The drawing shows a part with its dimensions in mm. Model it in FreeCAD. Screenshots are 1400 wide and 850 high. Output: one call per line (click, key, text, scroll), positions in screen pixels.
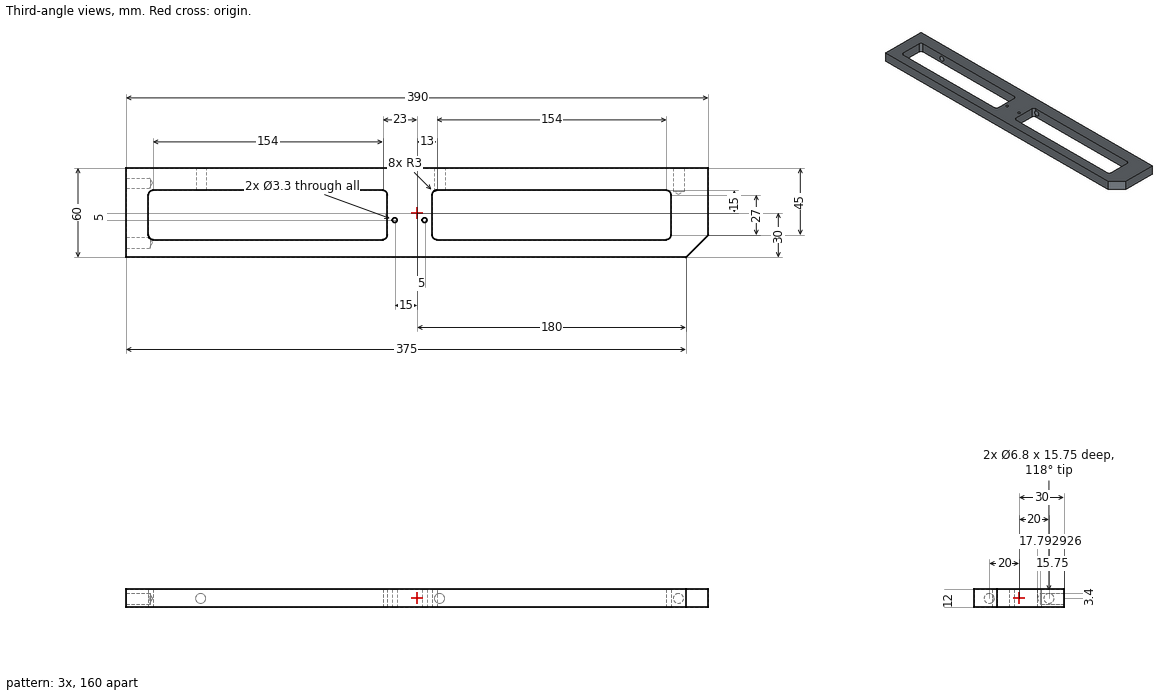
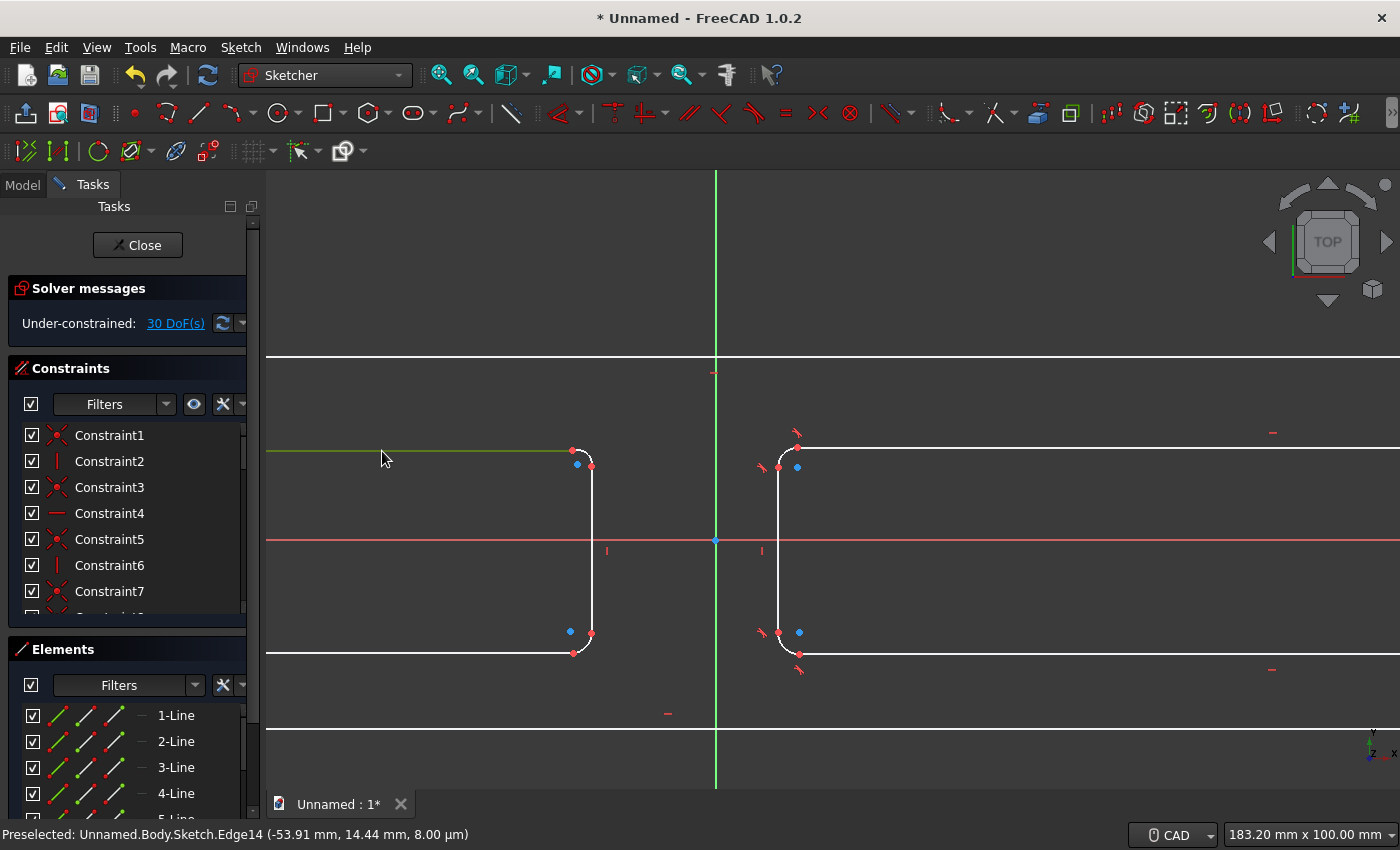
click(587, 453)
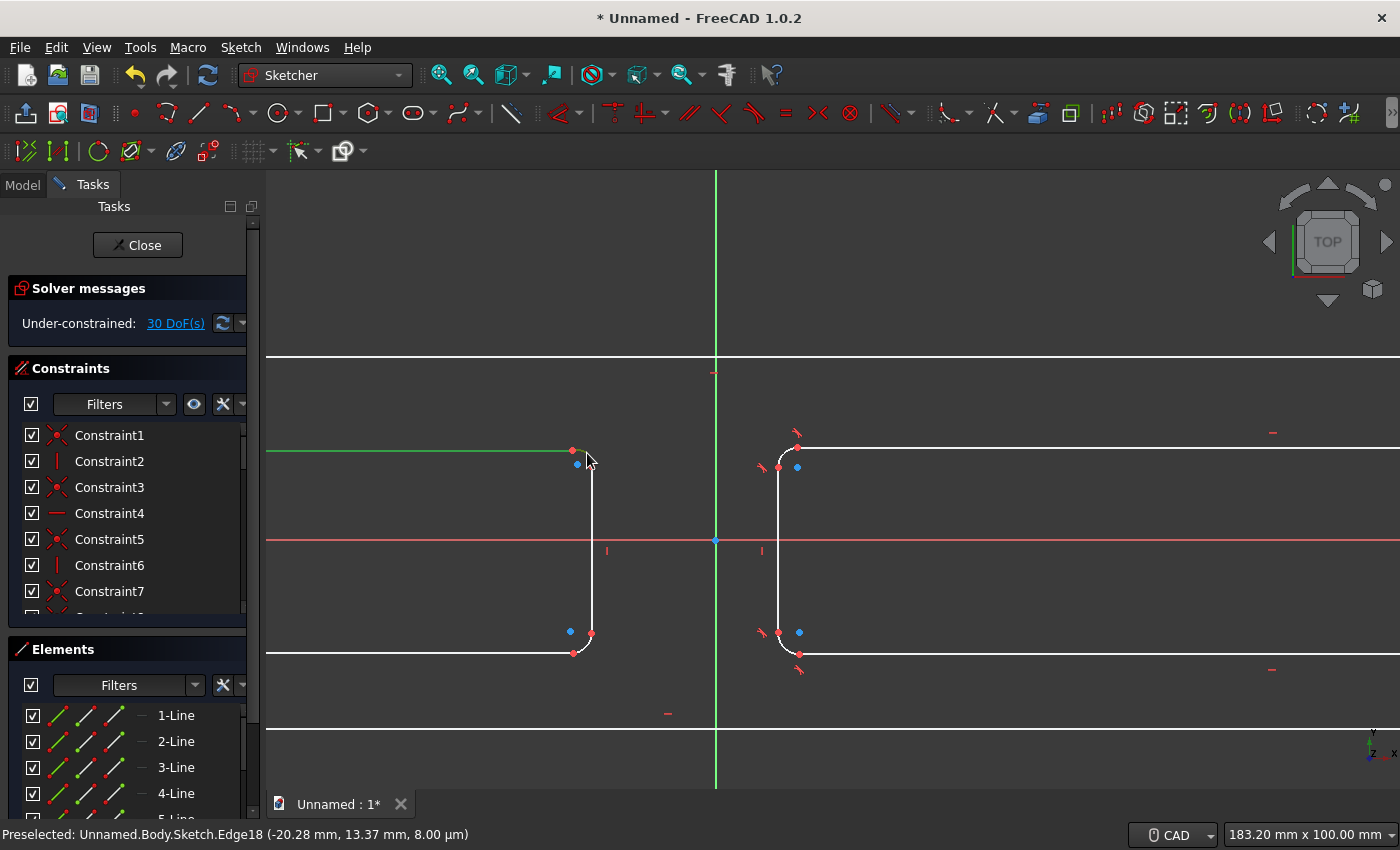
click(754, 114)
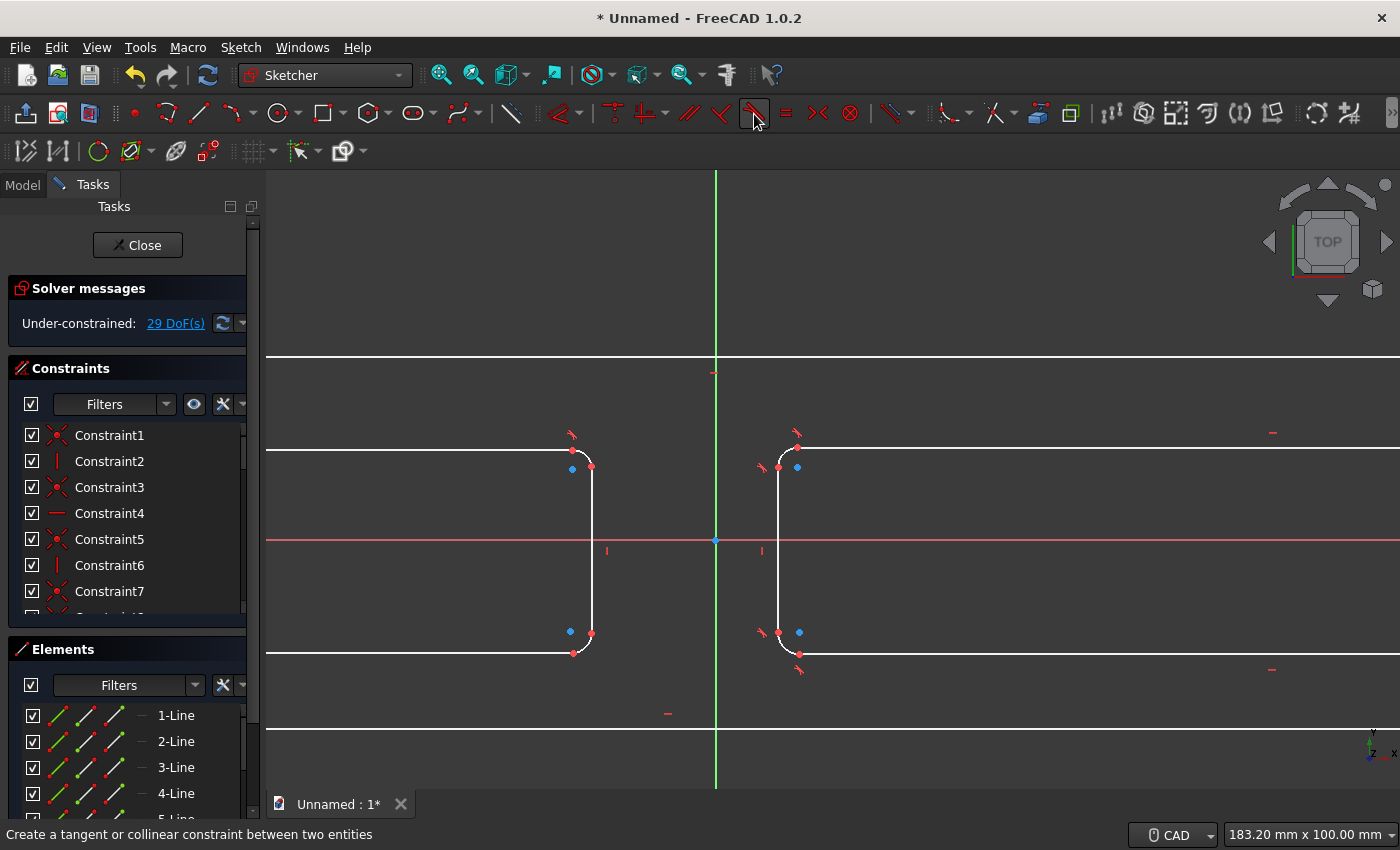
click(382, 450)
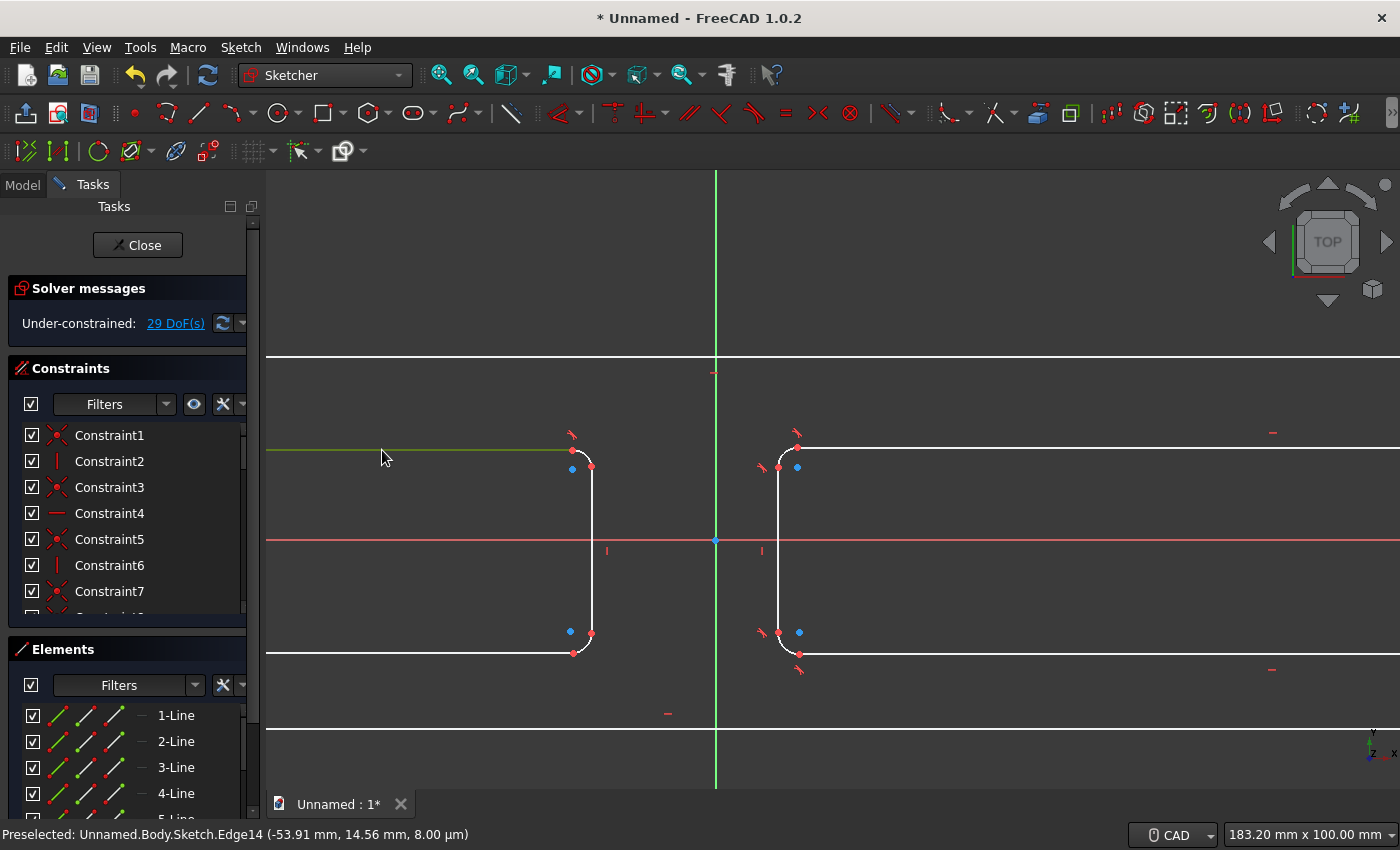
scroll(786, 453, down, 6)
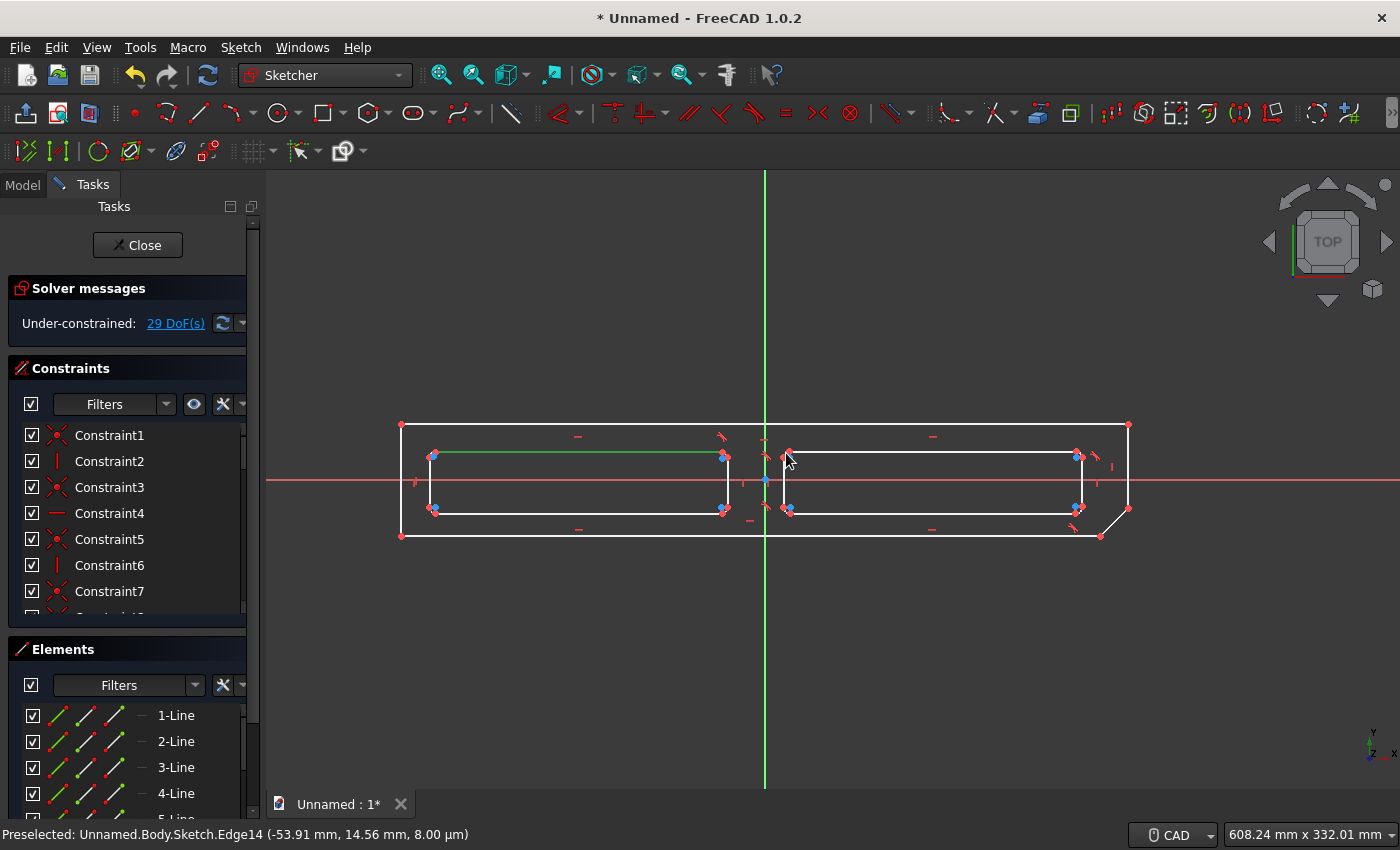
scroll(431, 454, up, 6)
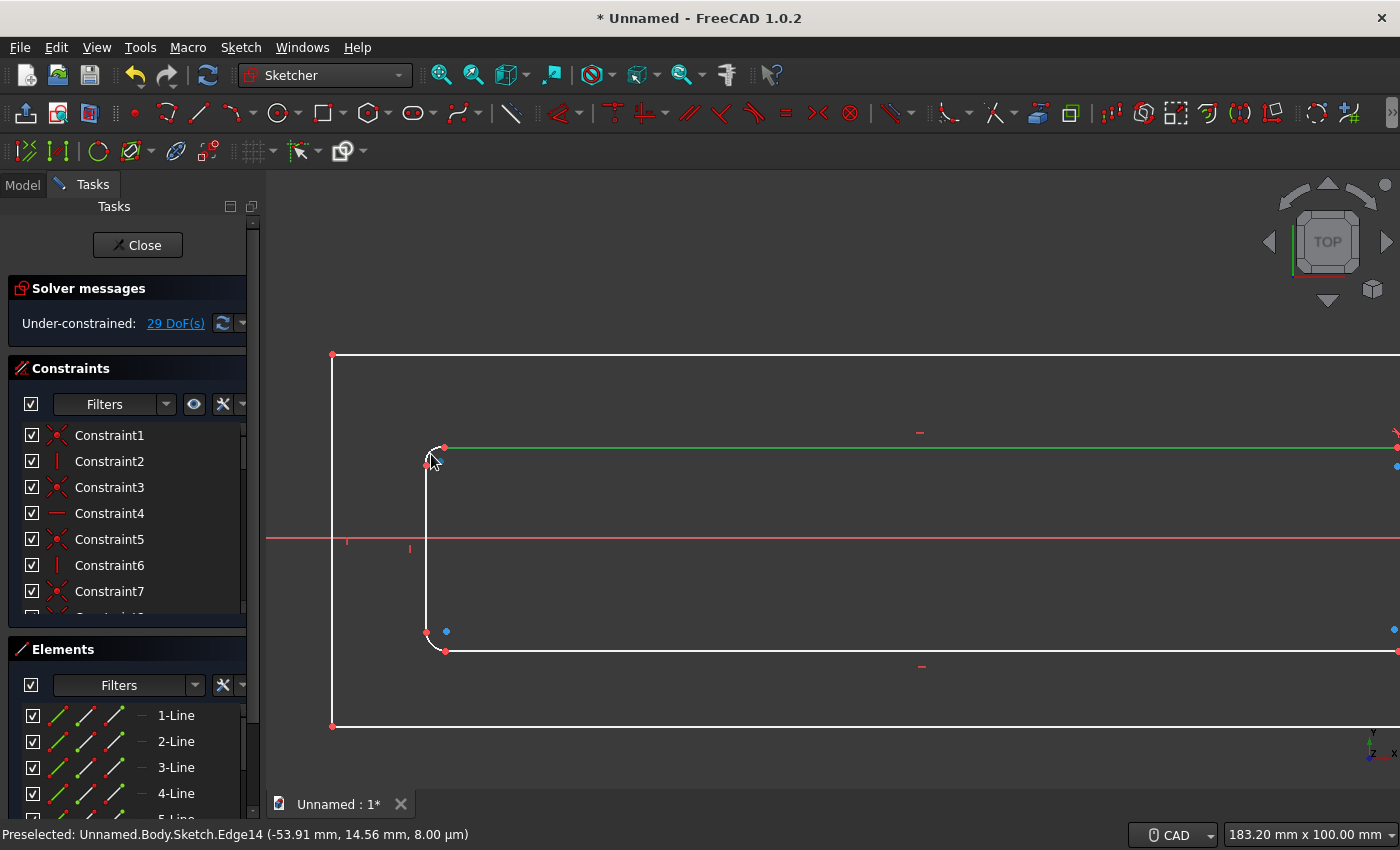
click(430, 451)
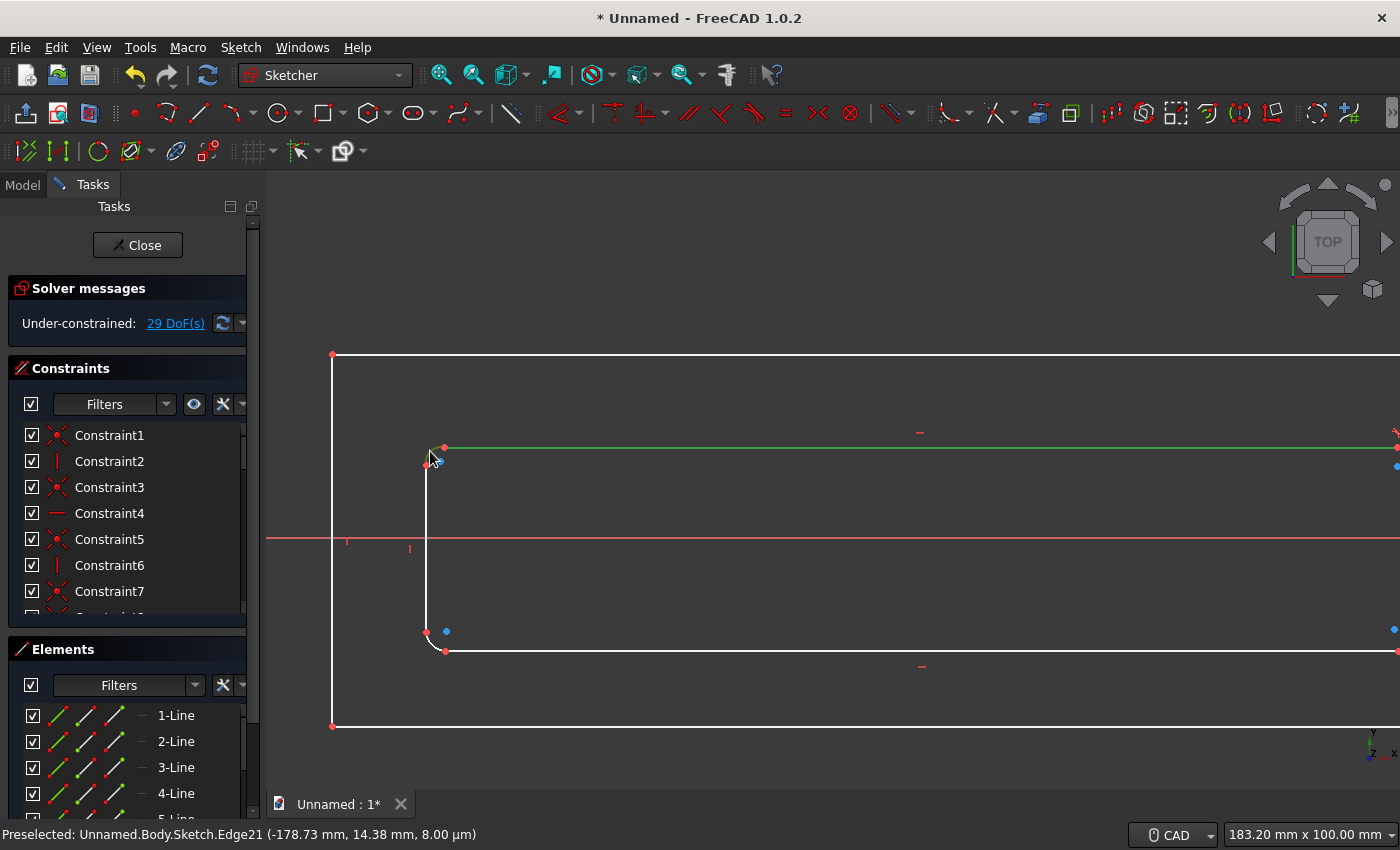
key(t)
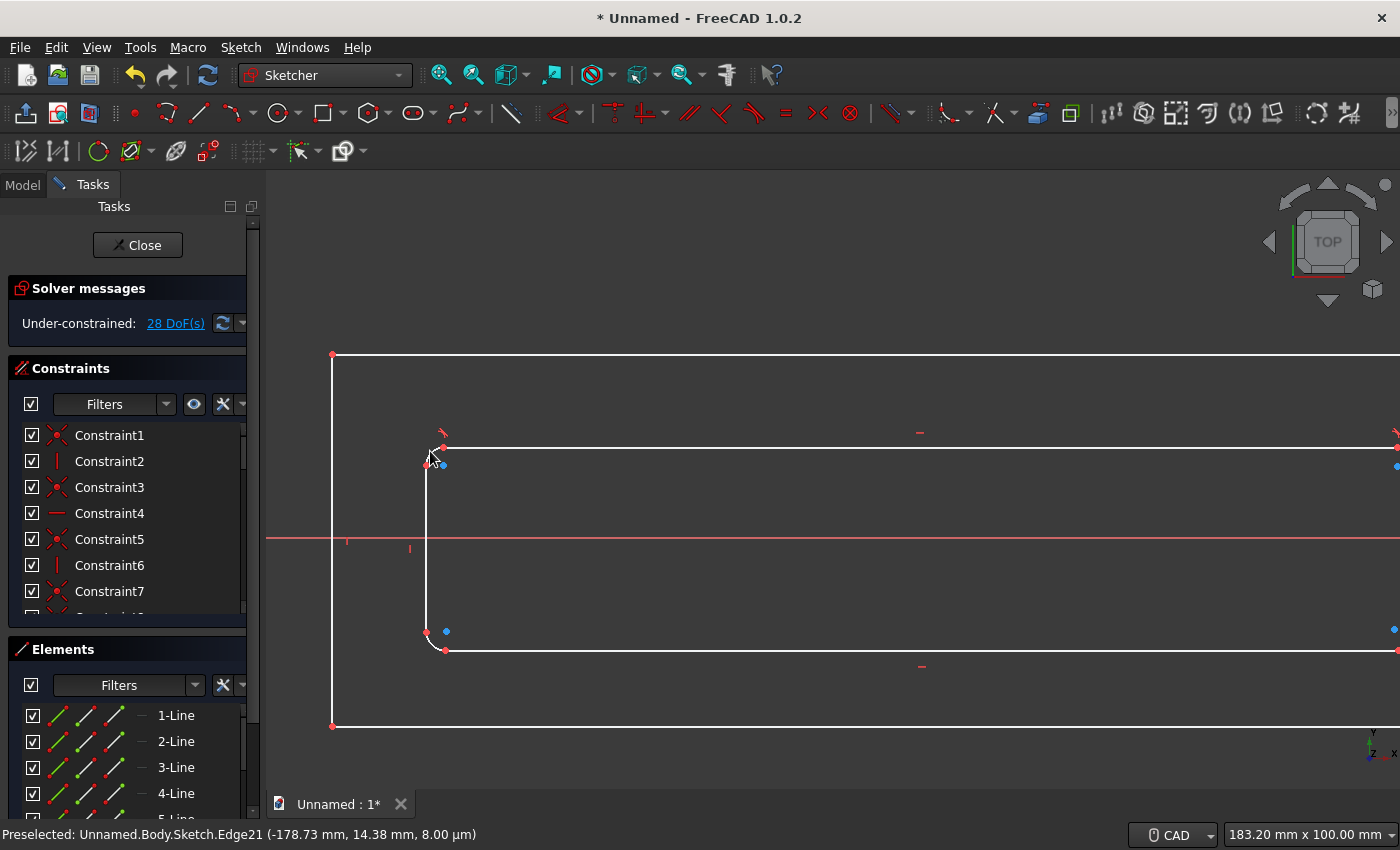
scroll(430, 454, down, 6)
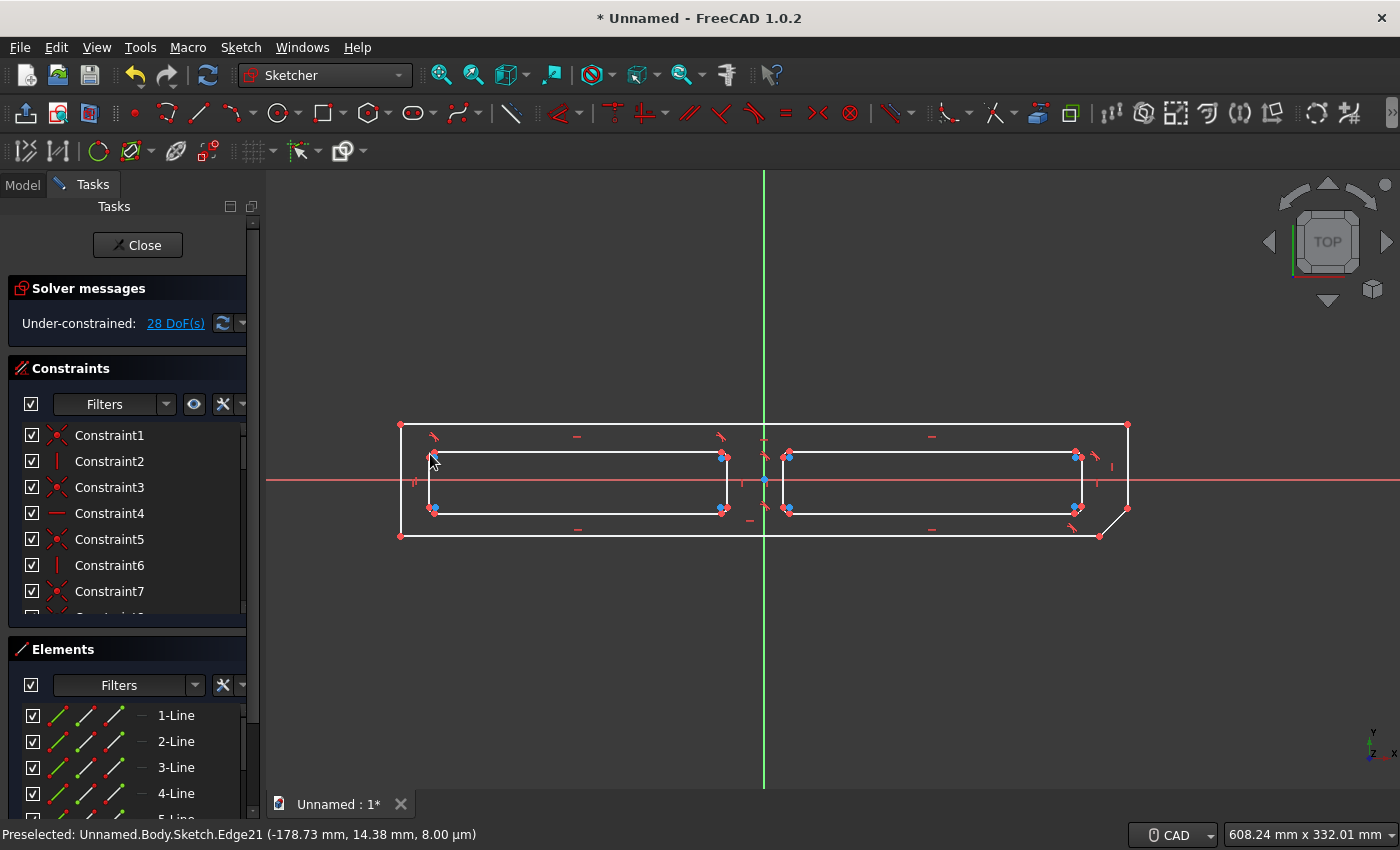
scroll(727, 473, up, 4)